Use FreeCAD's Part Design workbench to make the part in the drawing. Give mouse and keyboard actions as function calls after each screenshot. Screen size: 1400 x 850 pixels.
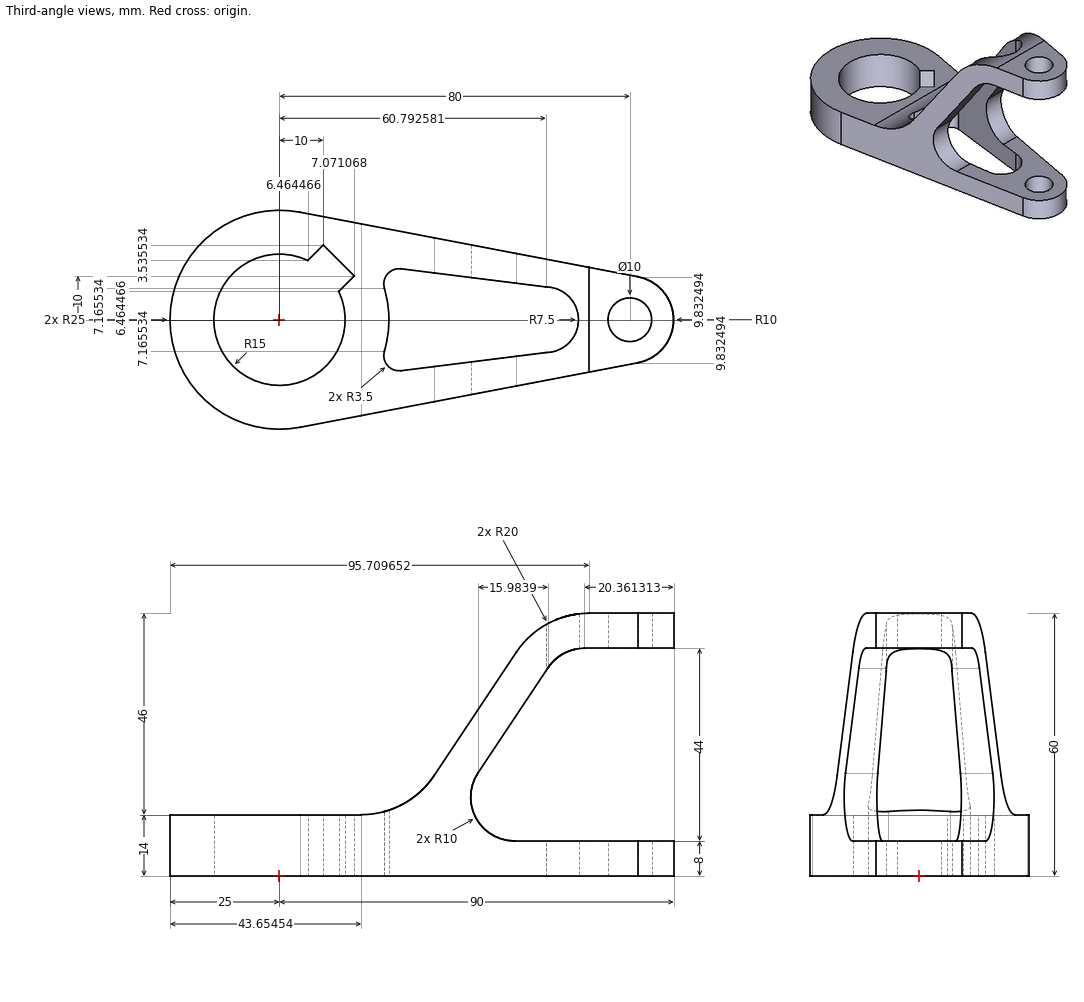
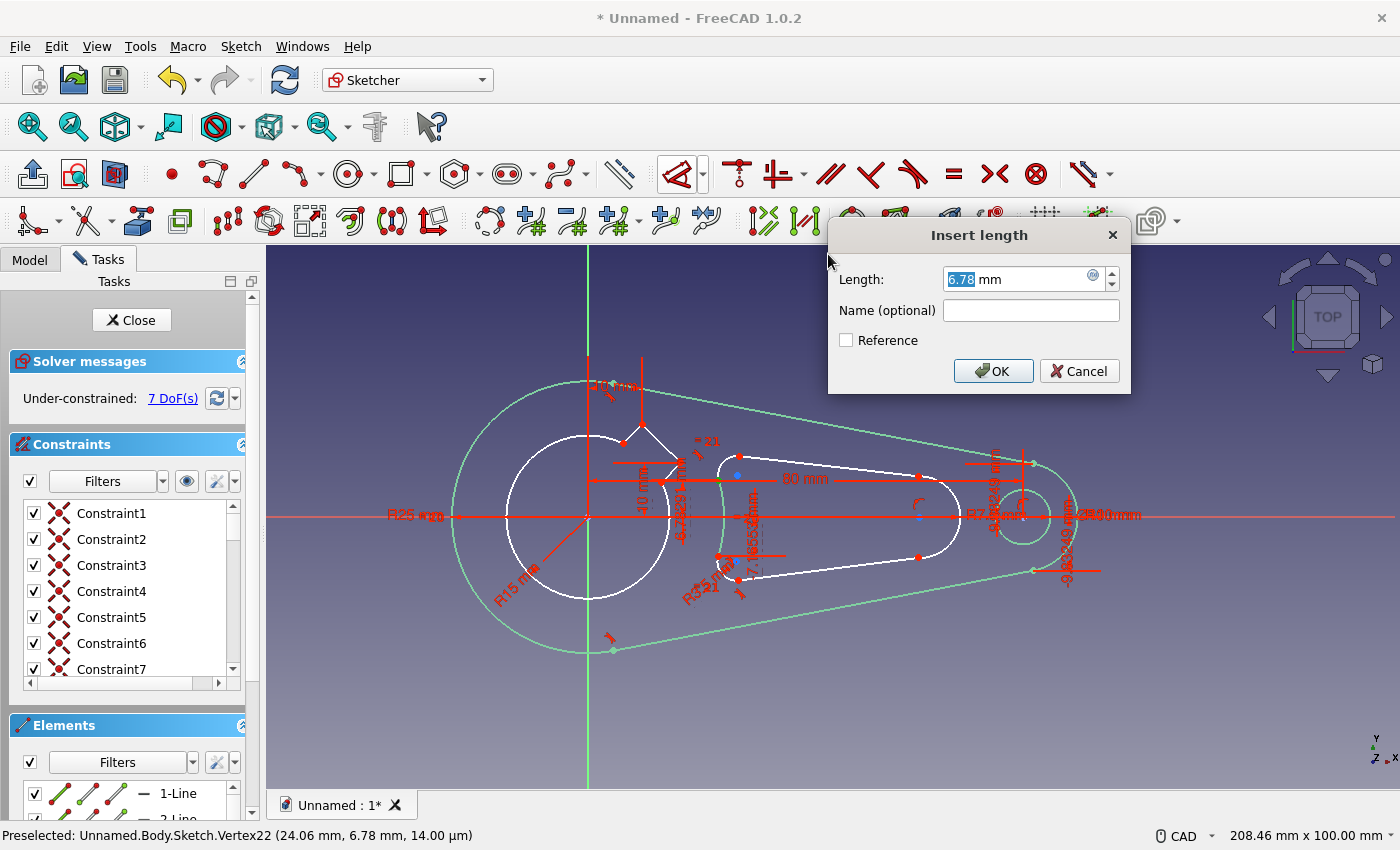
text(7.165534)
key(Return)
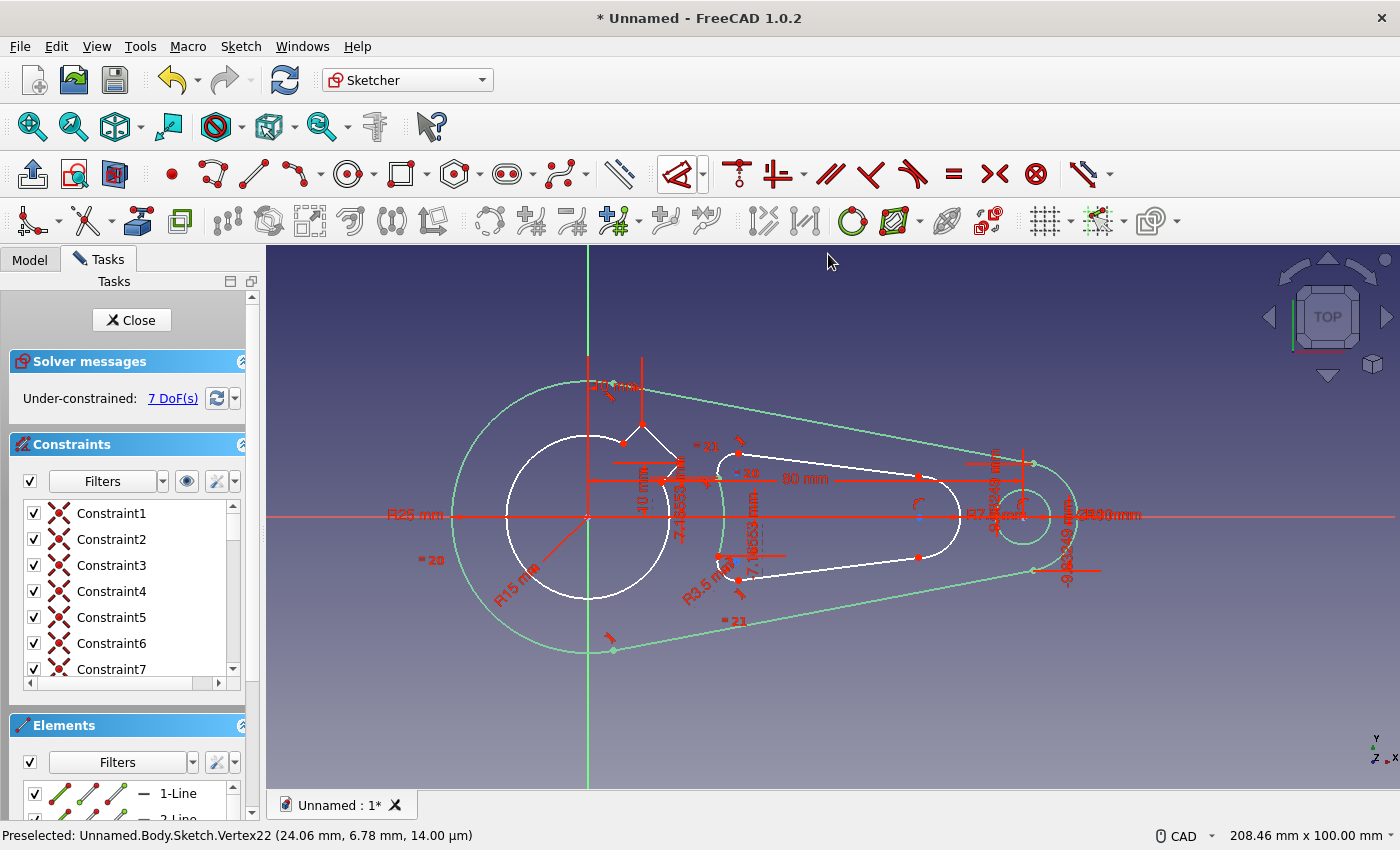
click(623, 444)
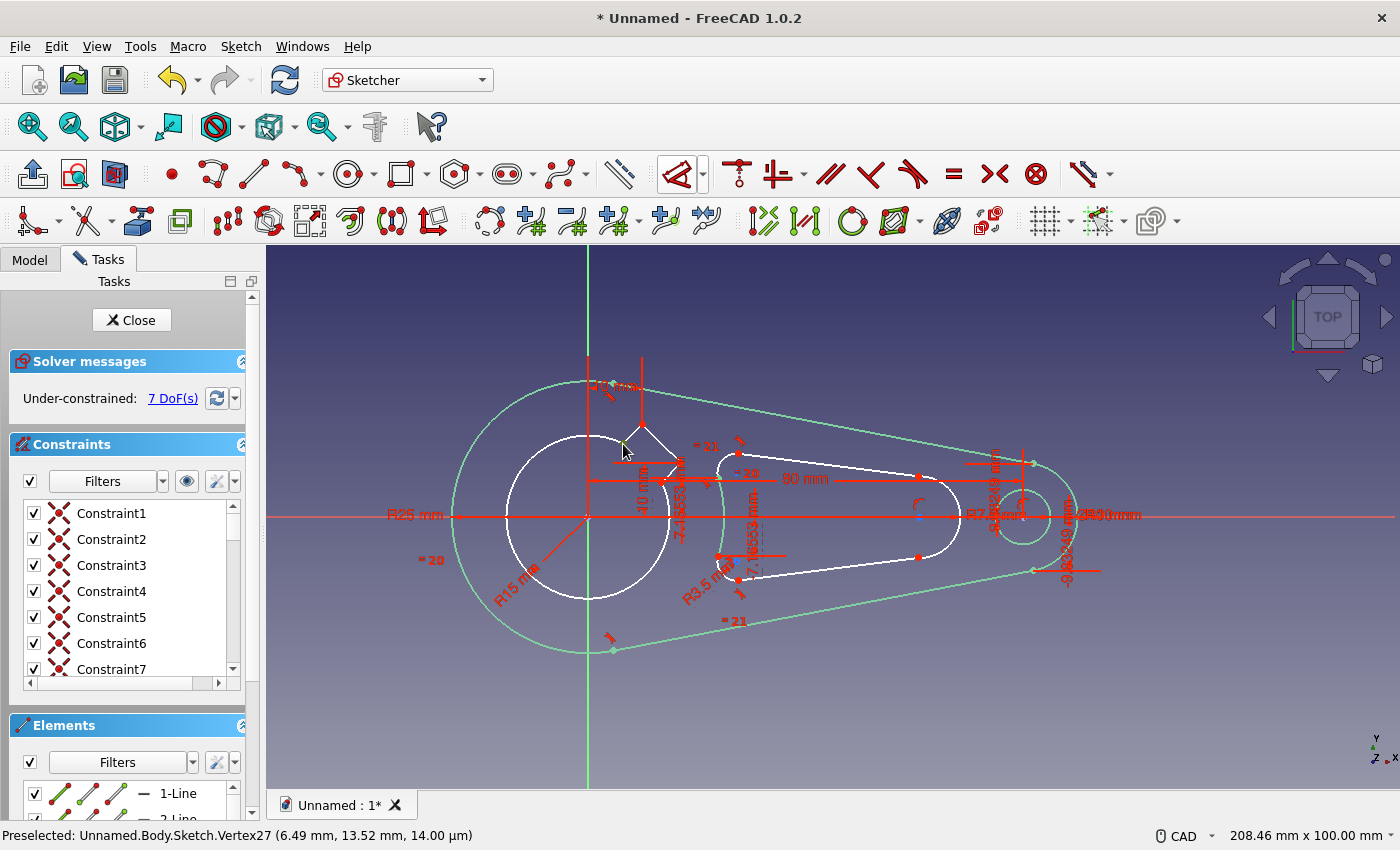
key(l)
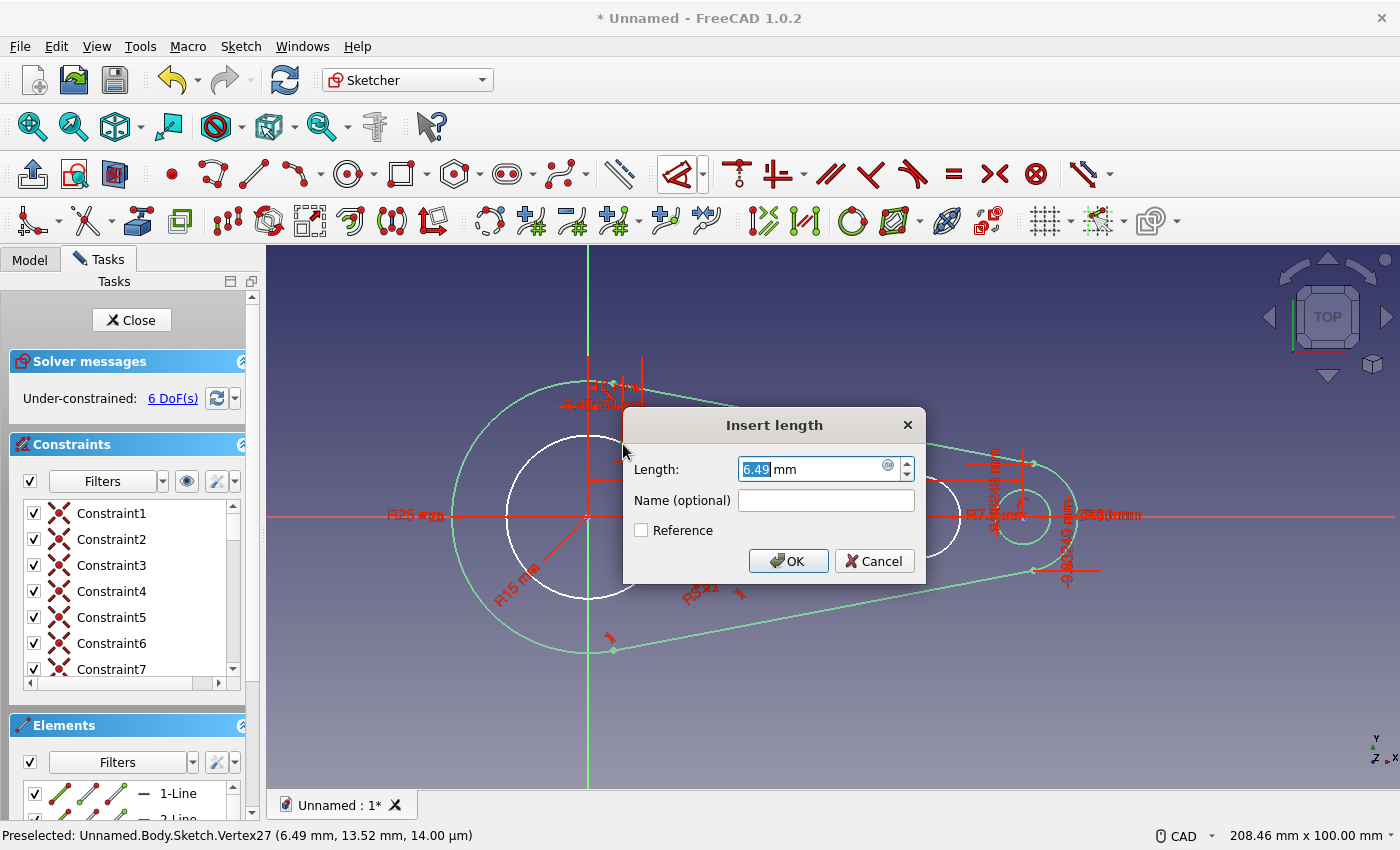
text(6.464466)
key(Return)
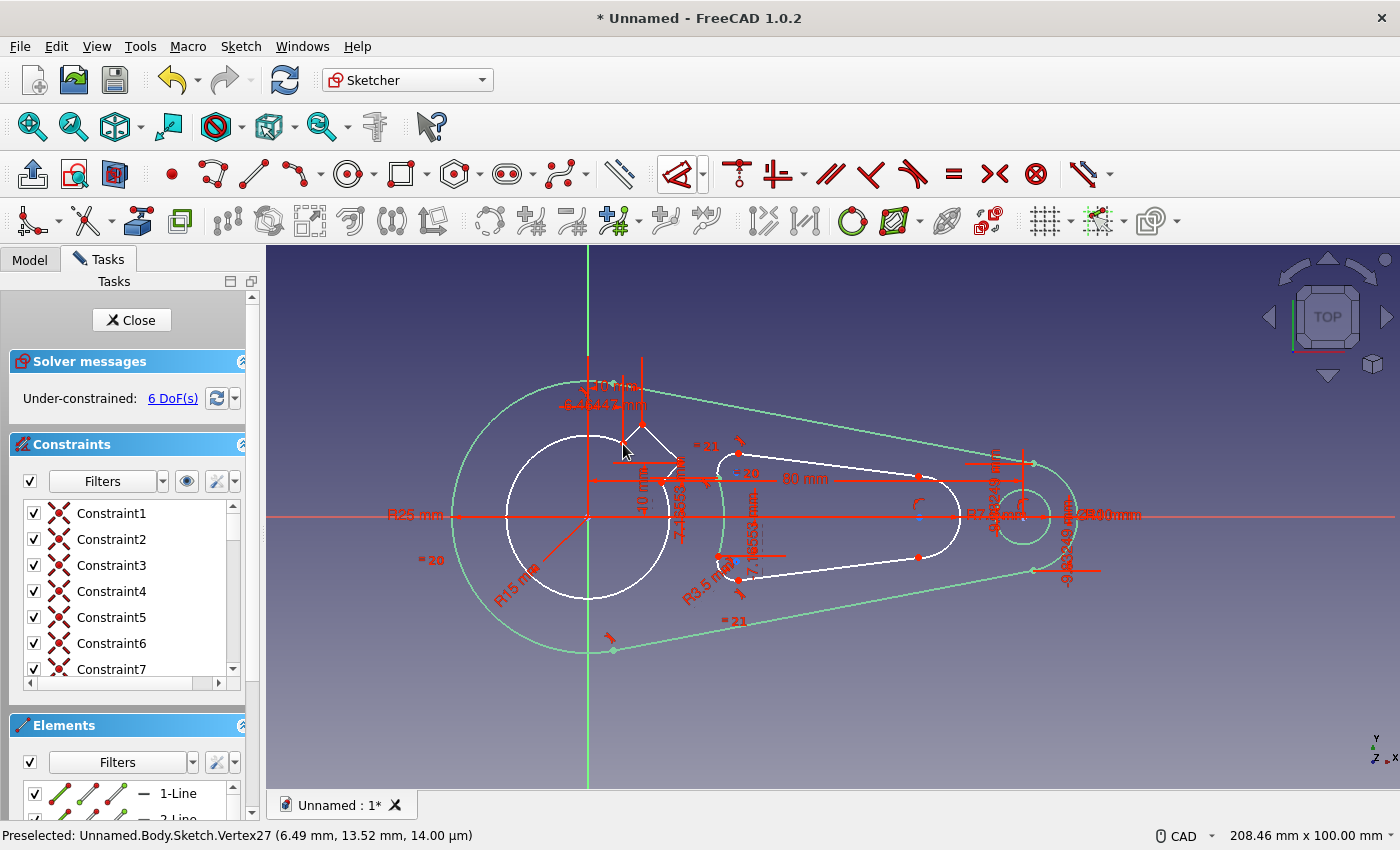
click(662, 483)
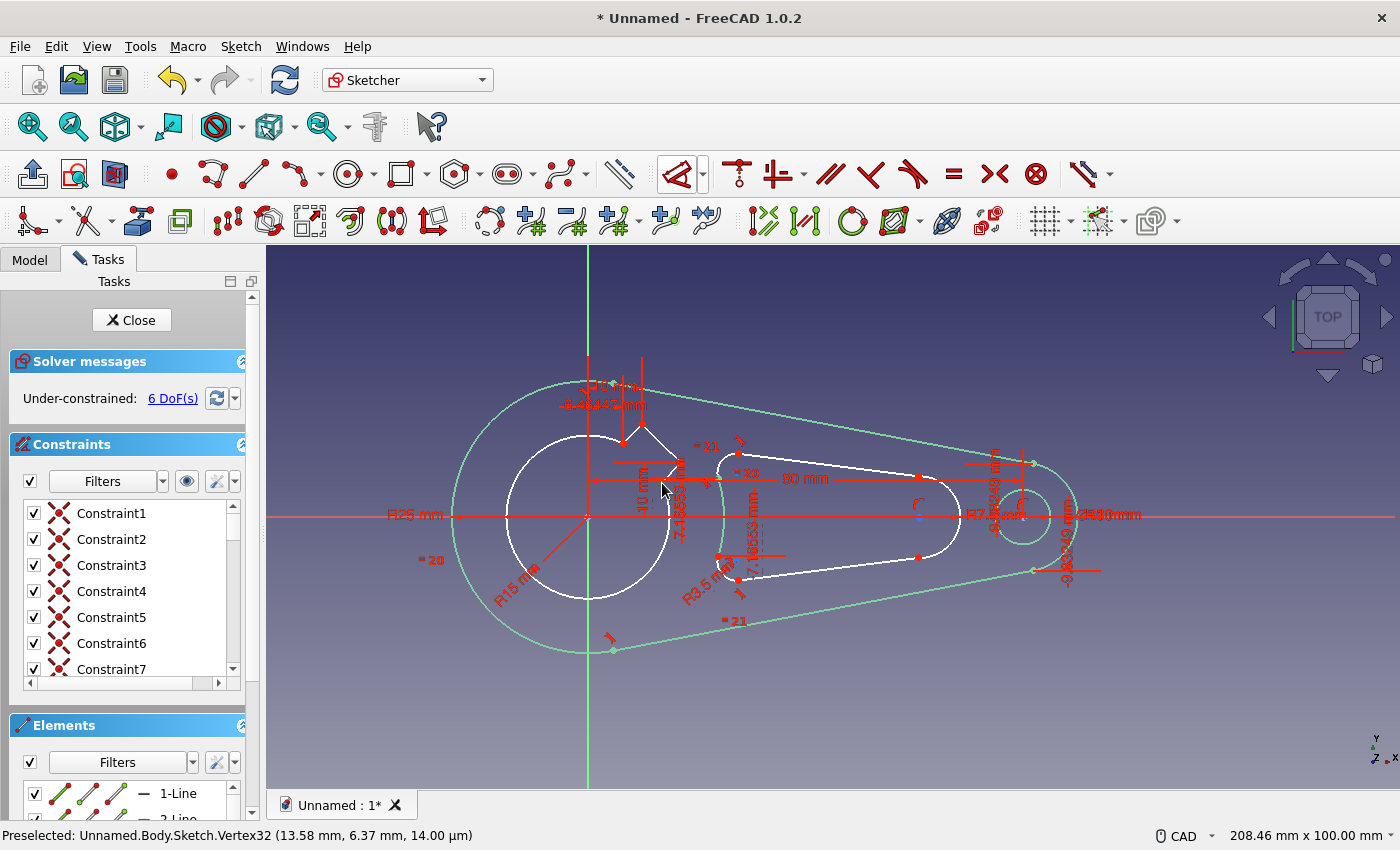
click(702, 174)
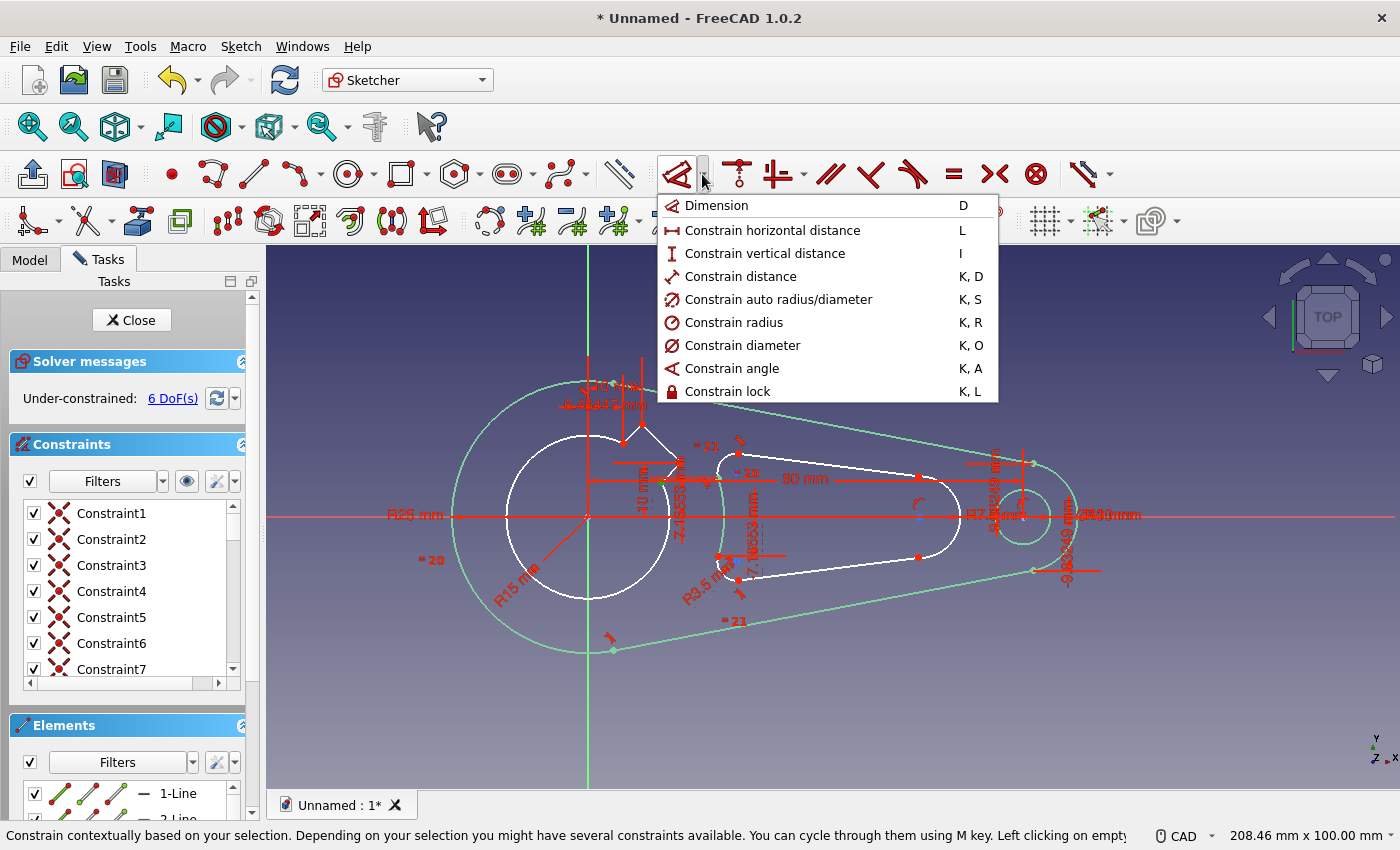
click(828, 254)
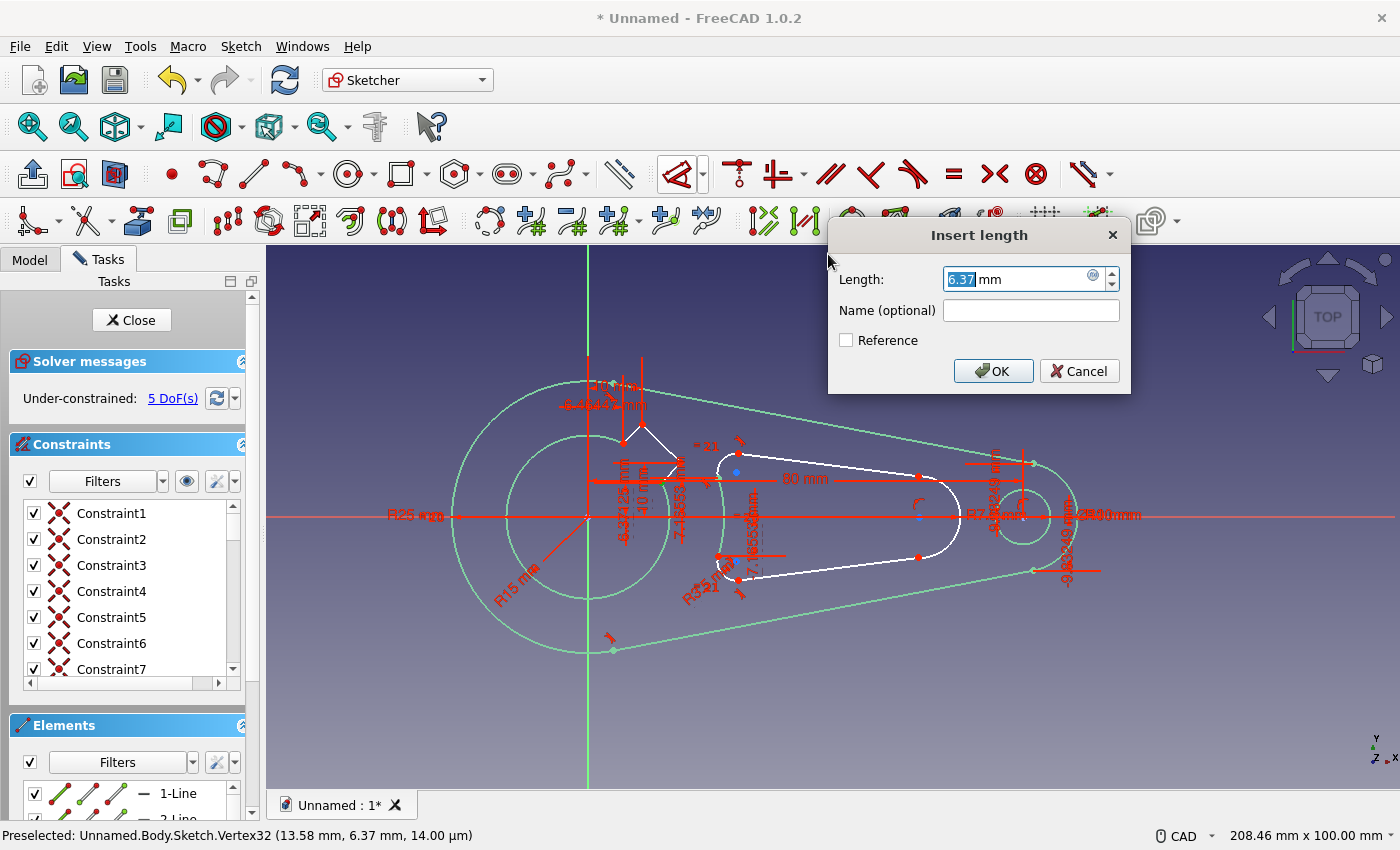
text(6.464466)
key(Return)